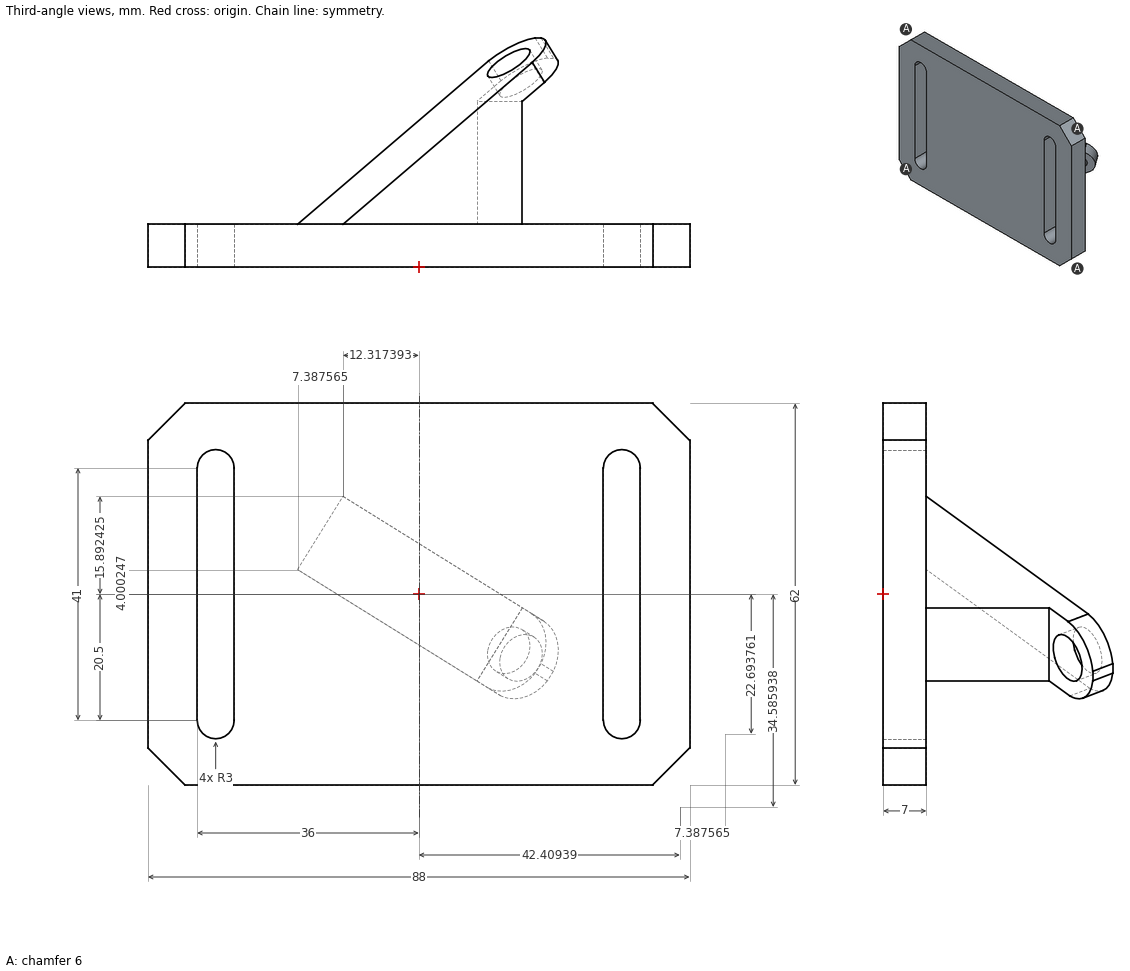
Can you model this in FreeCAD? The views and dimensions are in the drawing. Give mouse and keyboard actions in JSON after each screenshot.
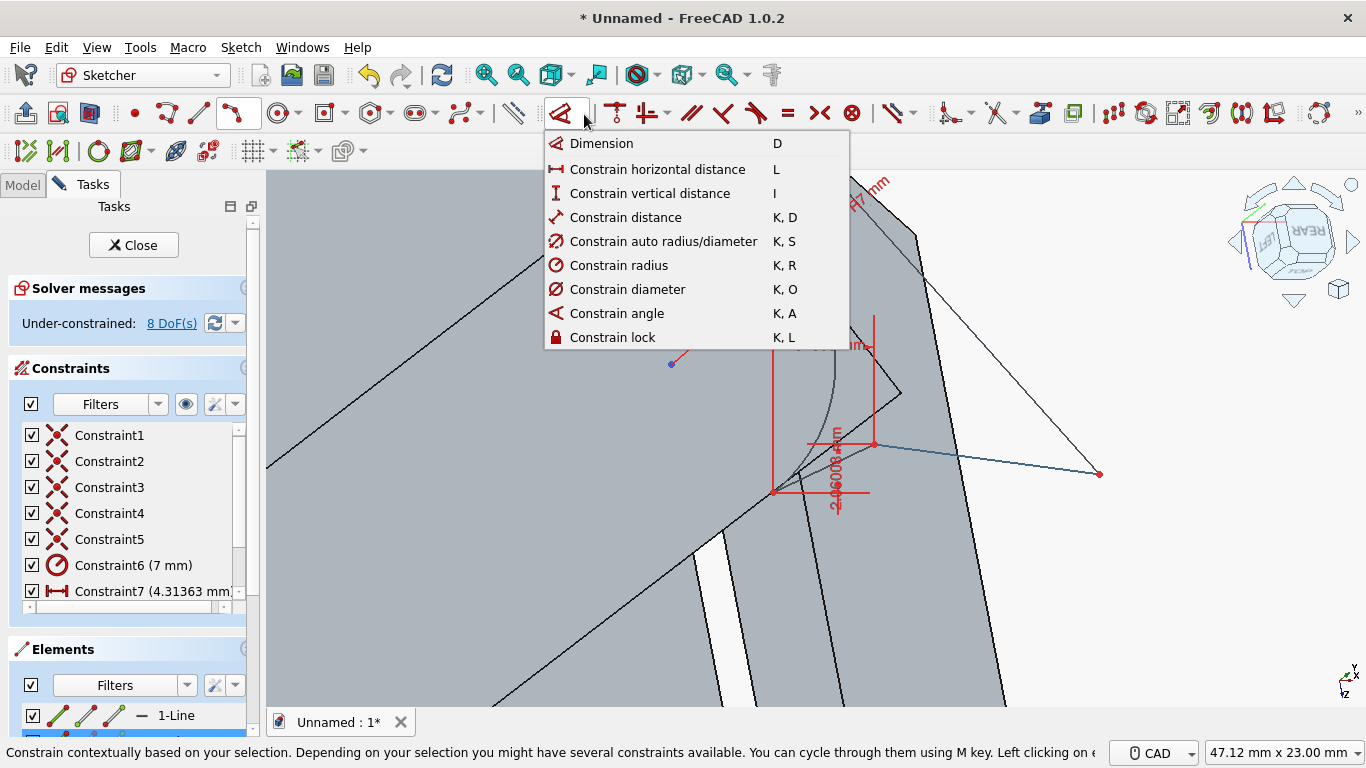
{"action": "left_click", "coordinate": [697, 169]}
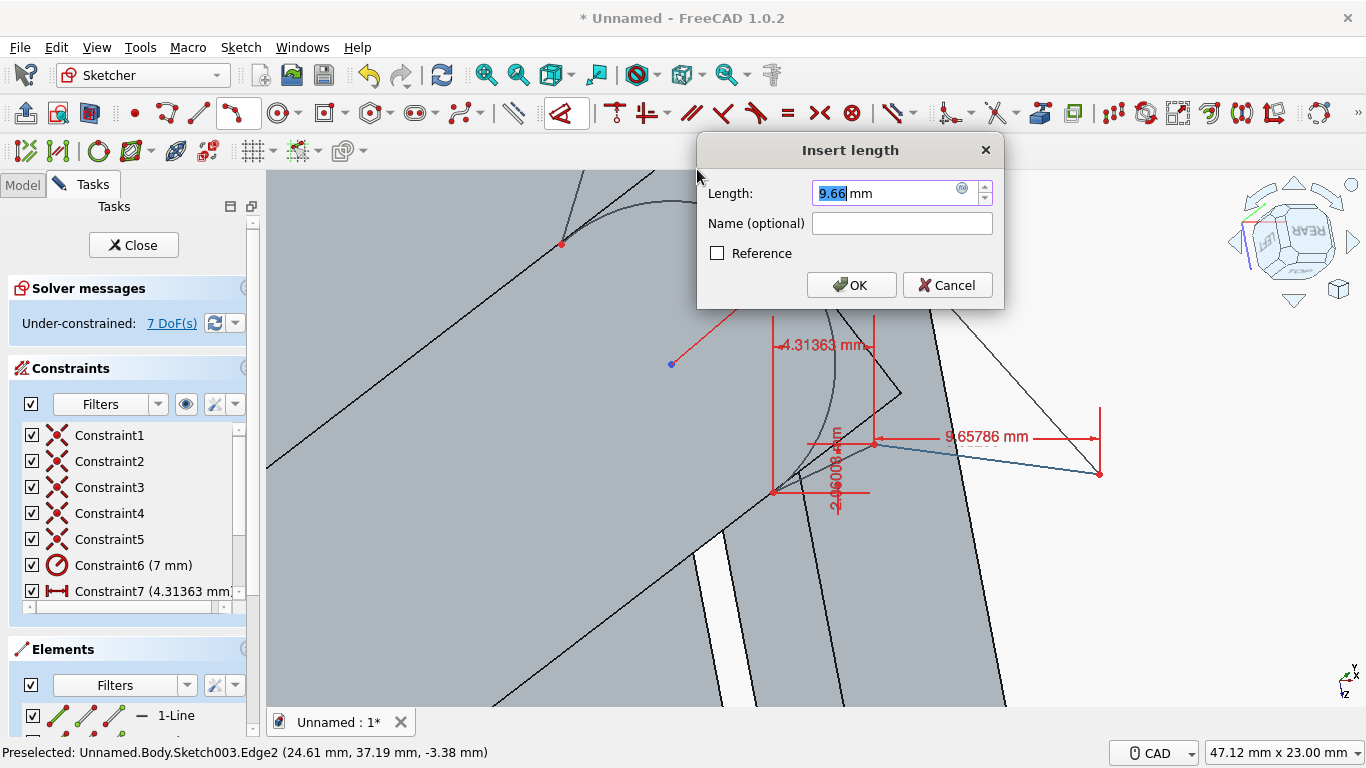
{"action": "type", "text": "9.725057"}
{"action": "key", "text": "Return"}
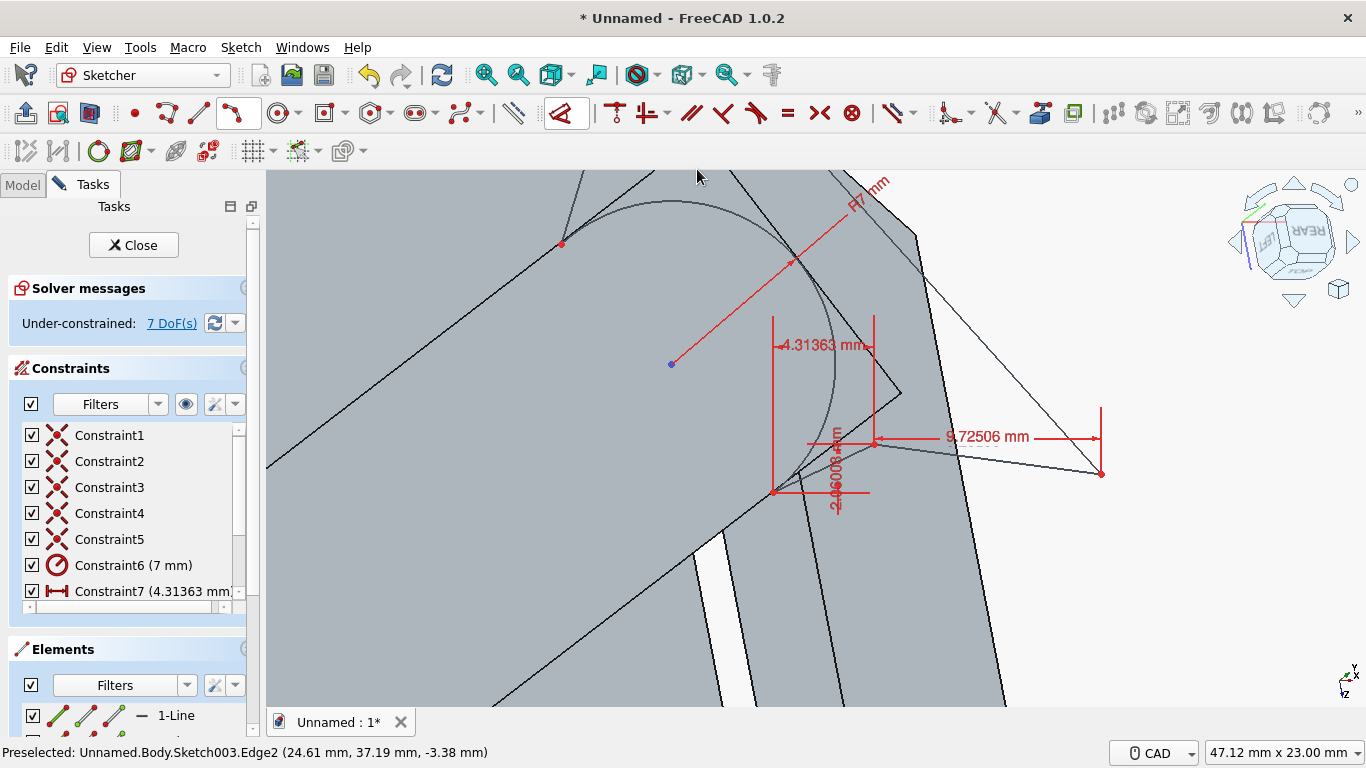
{"action": "scroll", "coordinate": [942, 453], "scroll_direction": "up", "scroll_amount": 2}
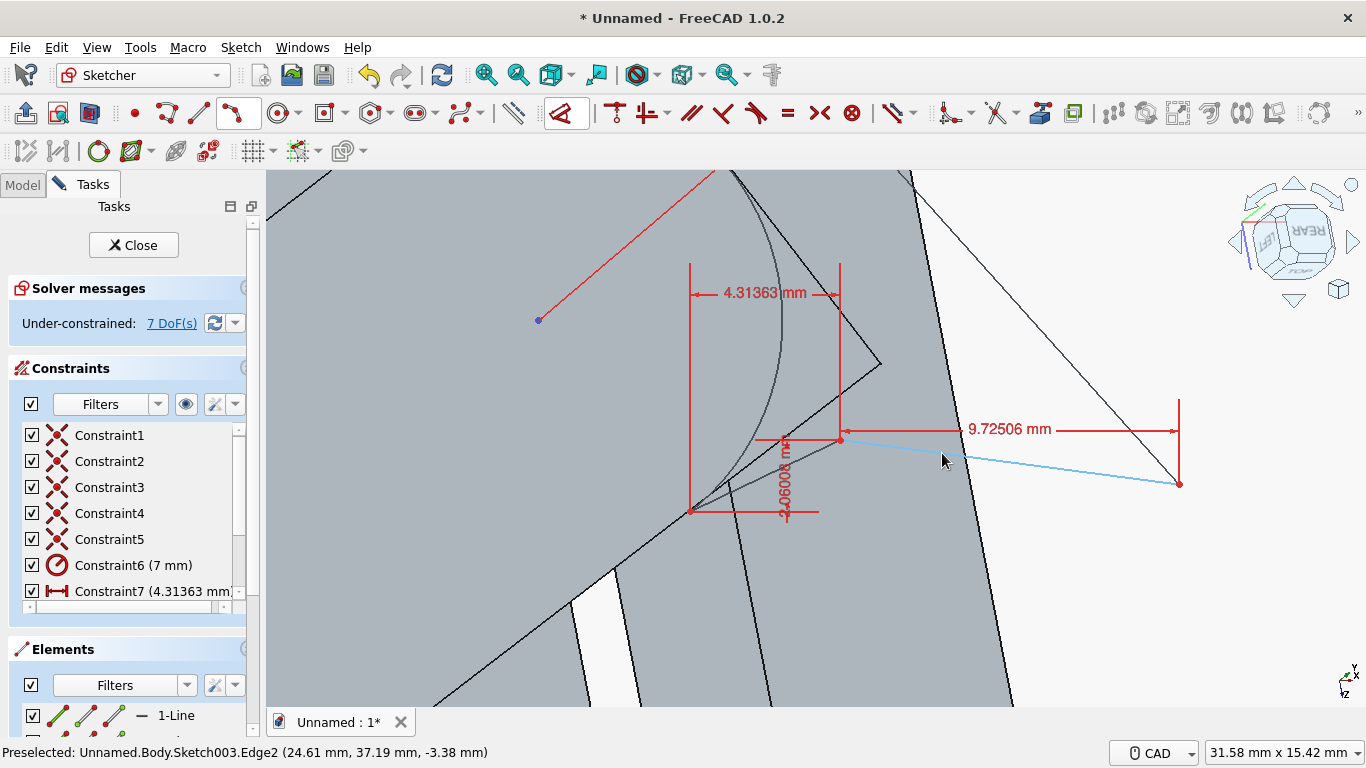
{"action": "left_click", "coordinate": [942, 453]}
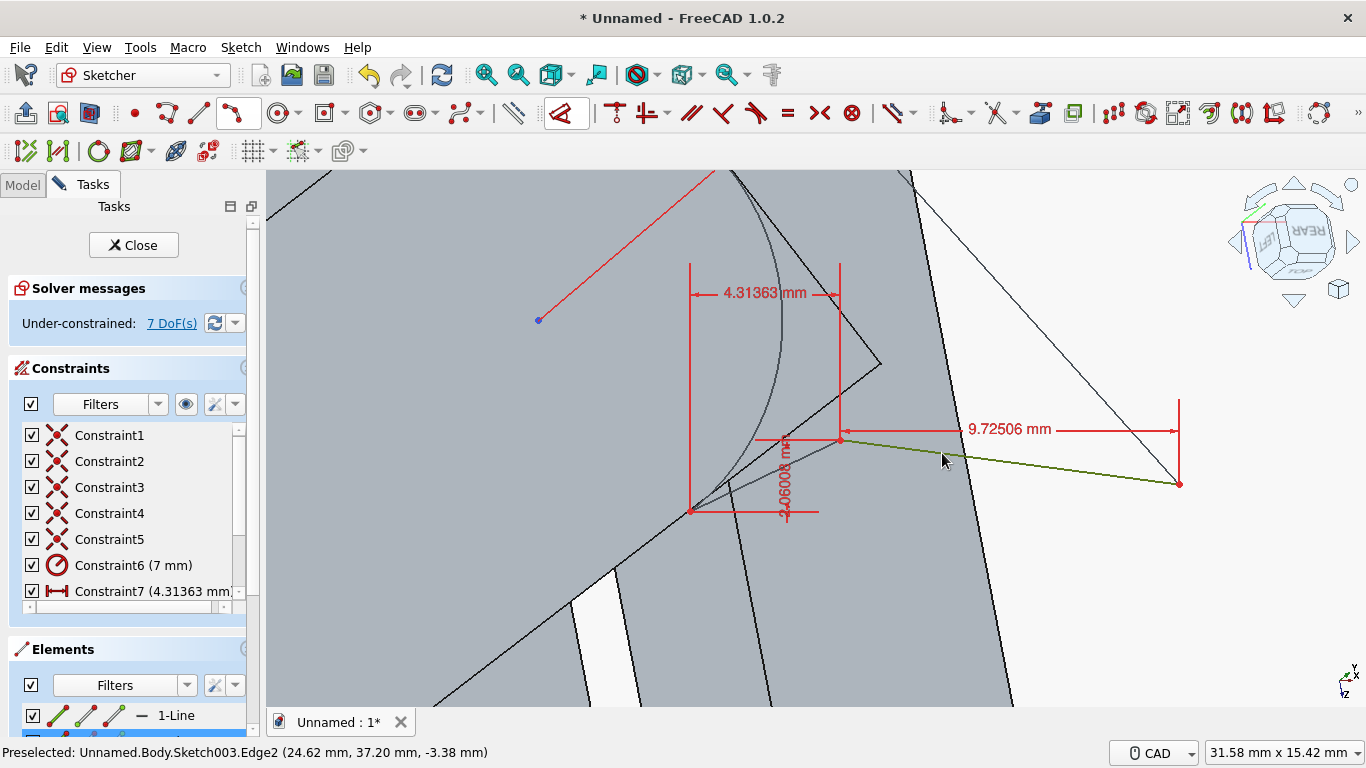
{"action": "key", "text": "i"}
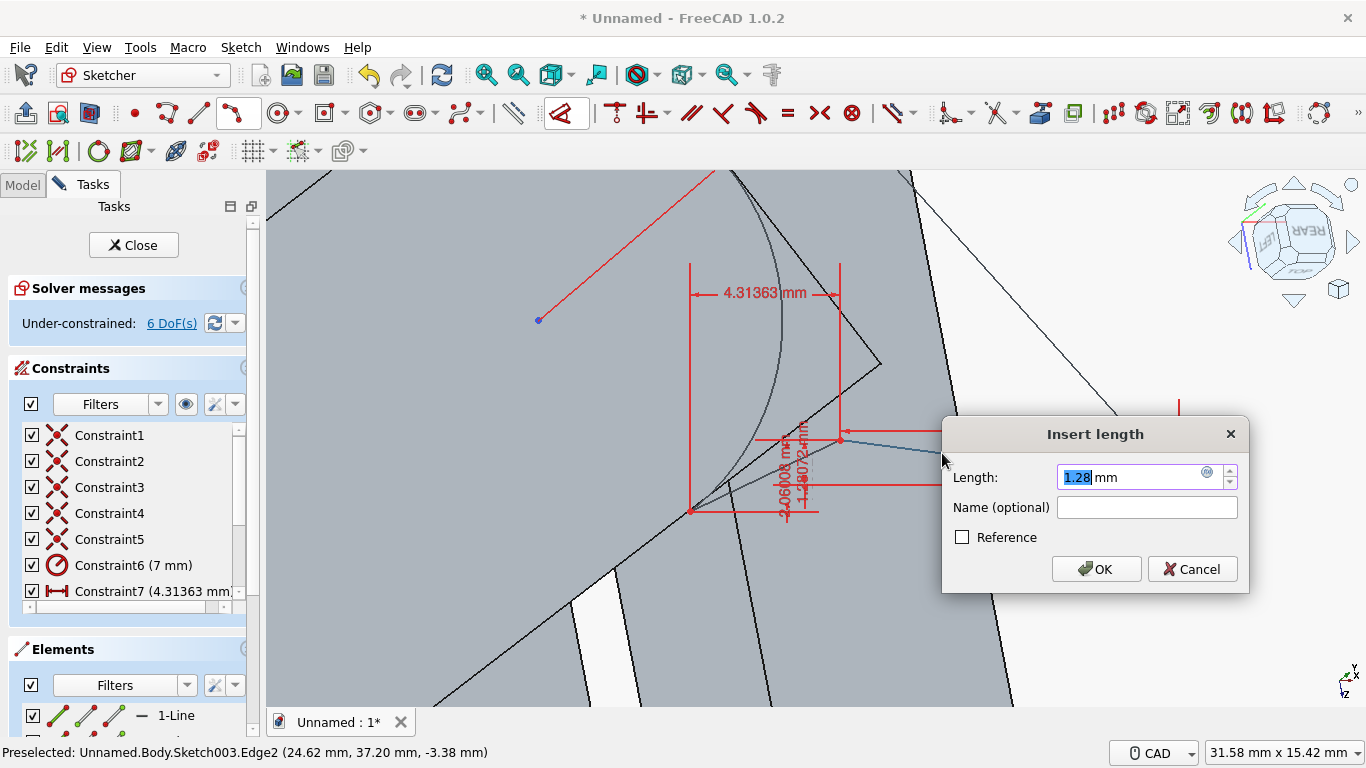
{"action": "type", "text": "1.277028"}
{"action": "key", "text": "Return"}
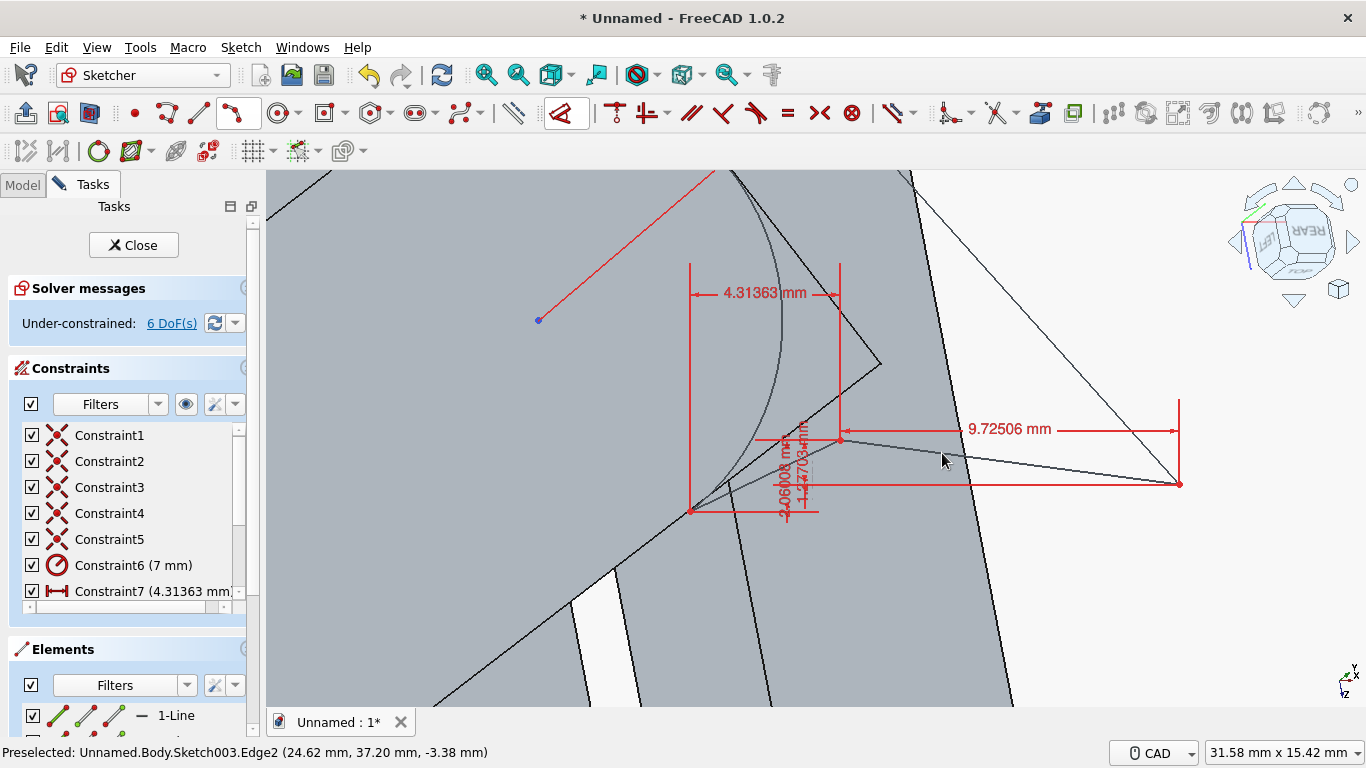
{"action": "scroll", "coordinate": [862, 459], "scroll_direction": "down", "scroll_amount": 7}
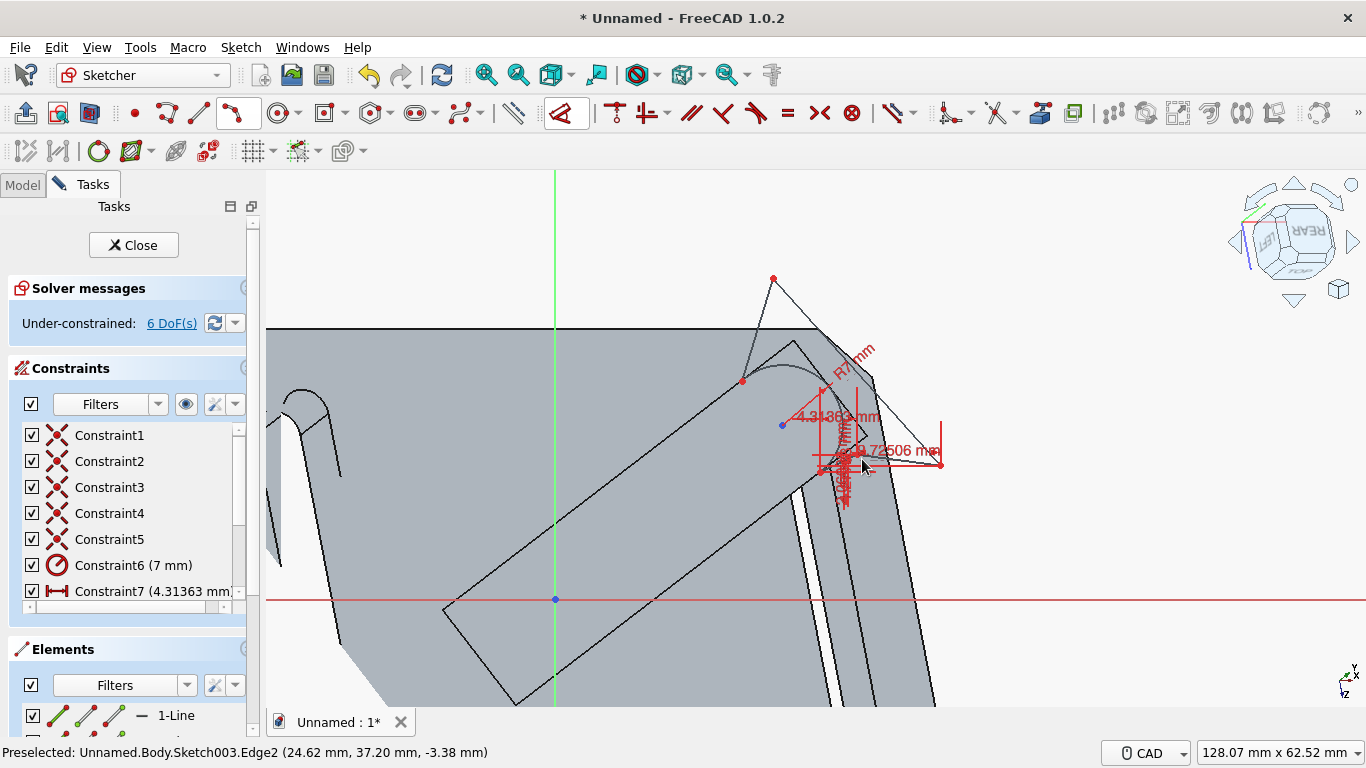
{"action": "scroll", "coordinate": [764, 309], "scroll_direction": "up", "scroll_amount": 2}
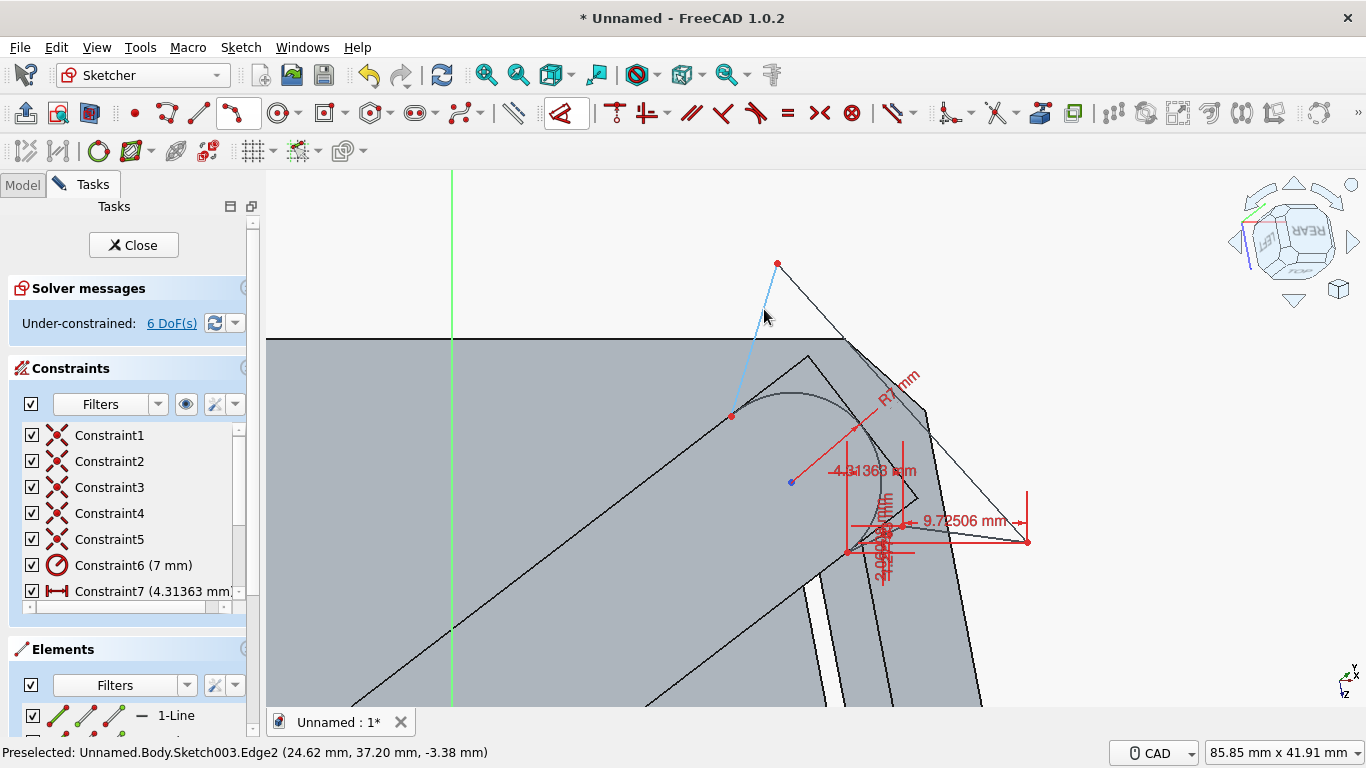
{"action": "left_click", "coordinate": [763, 309]}